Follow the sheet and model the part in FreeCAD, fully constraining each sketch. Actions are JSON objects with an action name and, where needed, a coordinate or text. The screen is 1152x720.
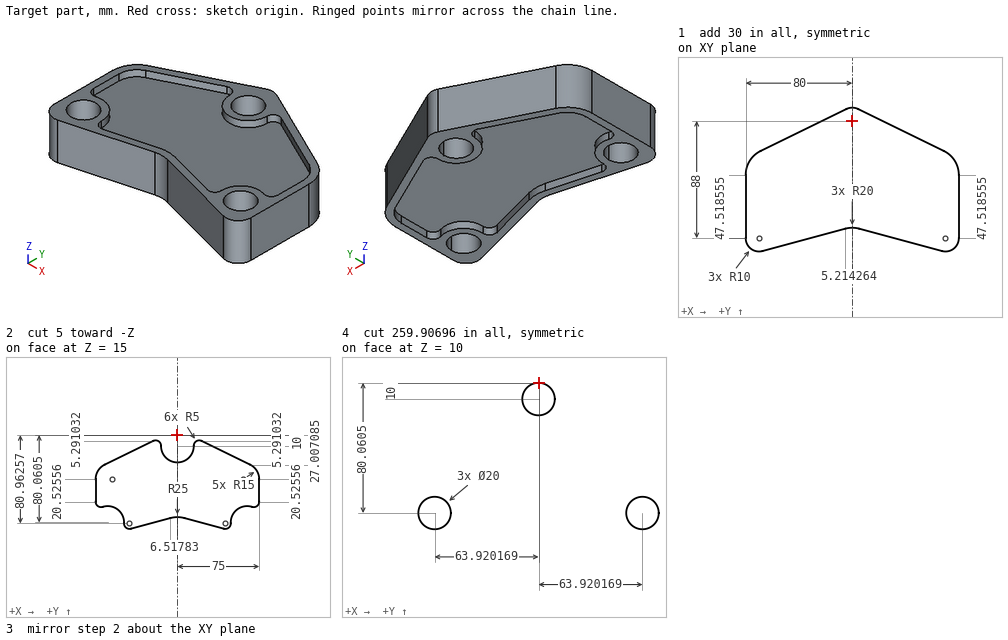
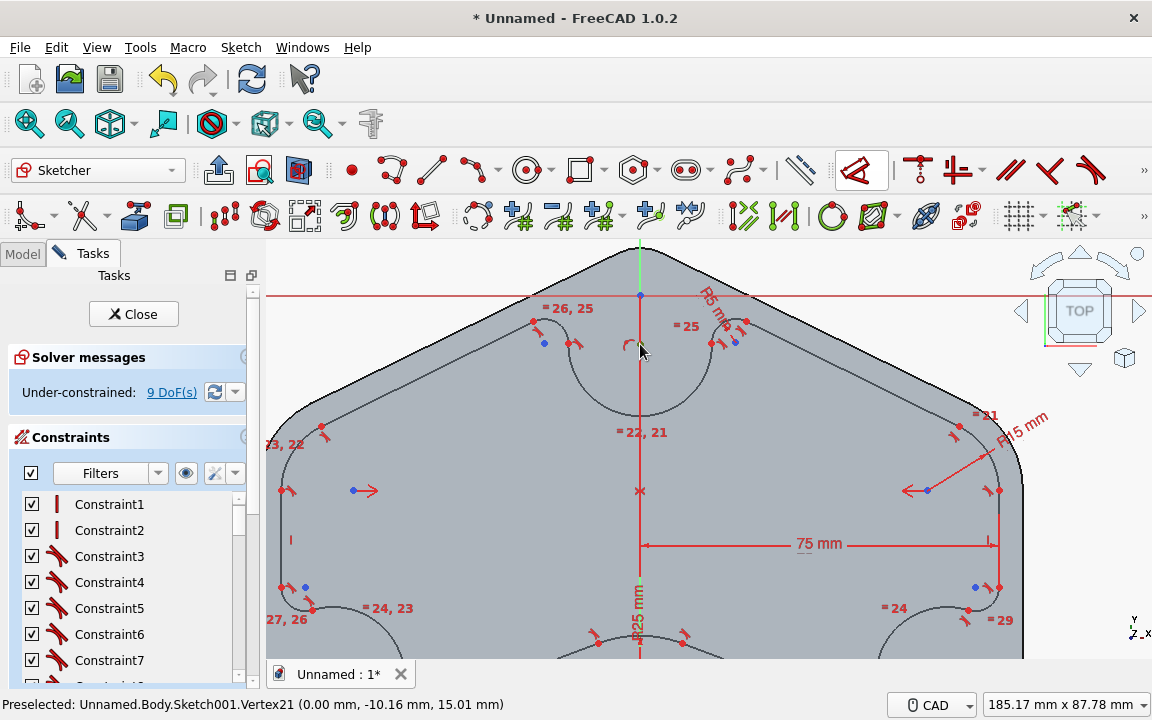
{"action": "left_click", "coordinate": [882, 170]}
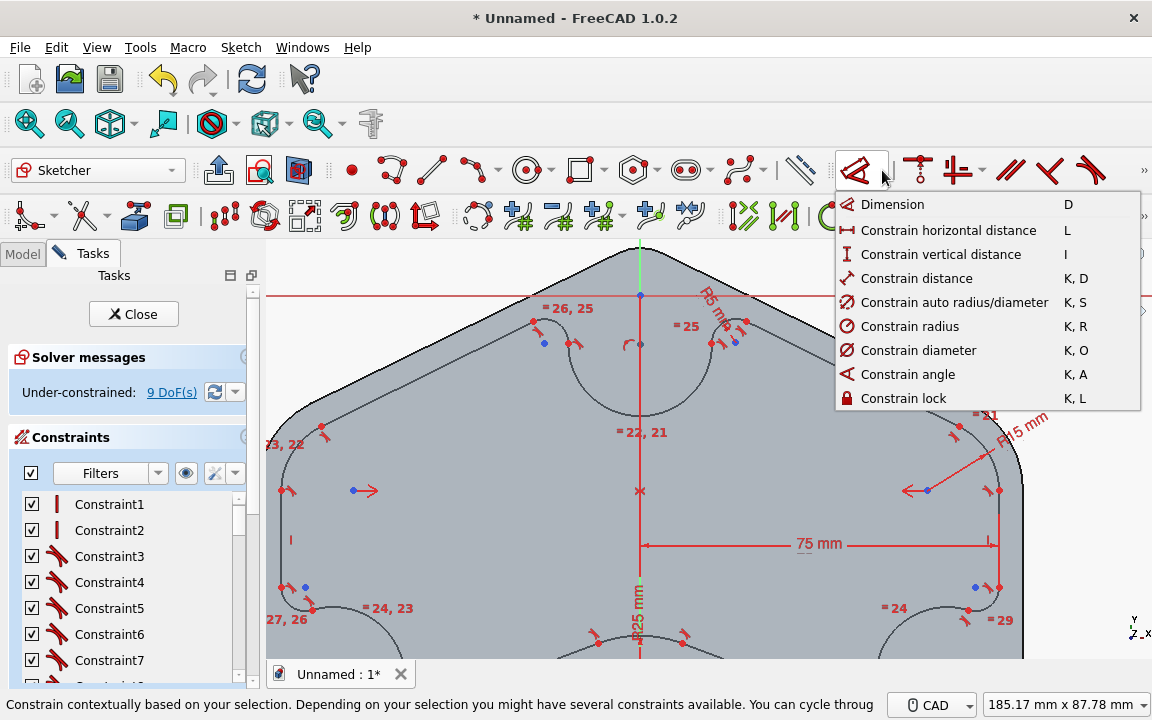
{"action": "left_click", "coordinate": [988, 254]}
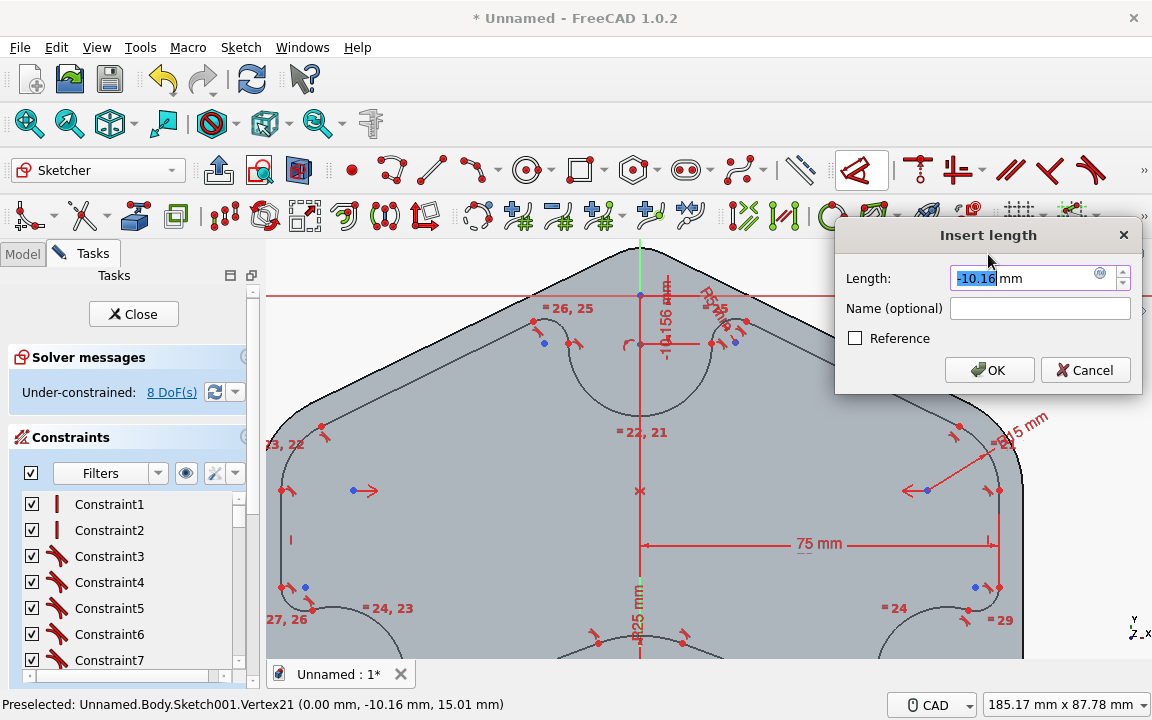
{"action": "type", "text": "-10"}
{"action": "key", "text": "Return"}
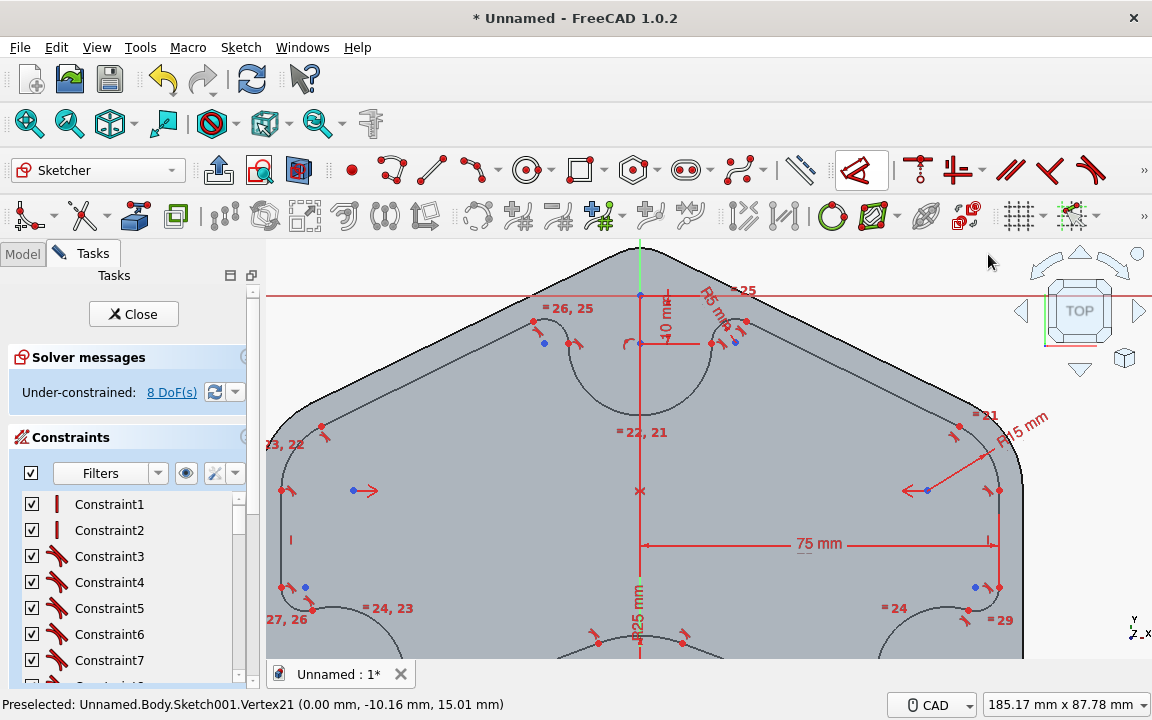
{"action": "scroll", "coordinate": [641, 343], "scroll_direction": "down", "scroll_amount": 2}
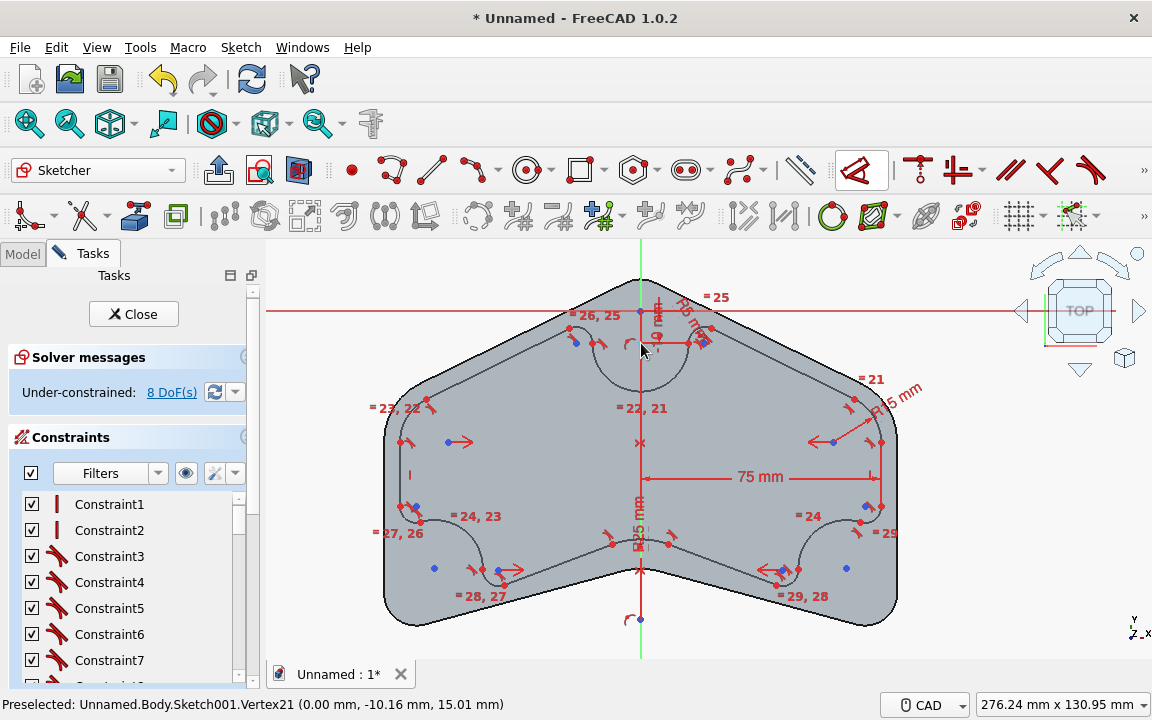
{"action": "left_click", "coordinate": [881, 487]}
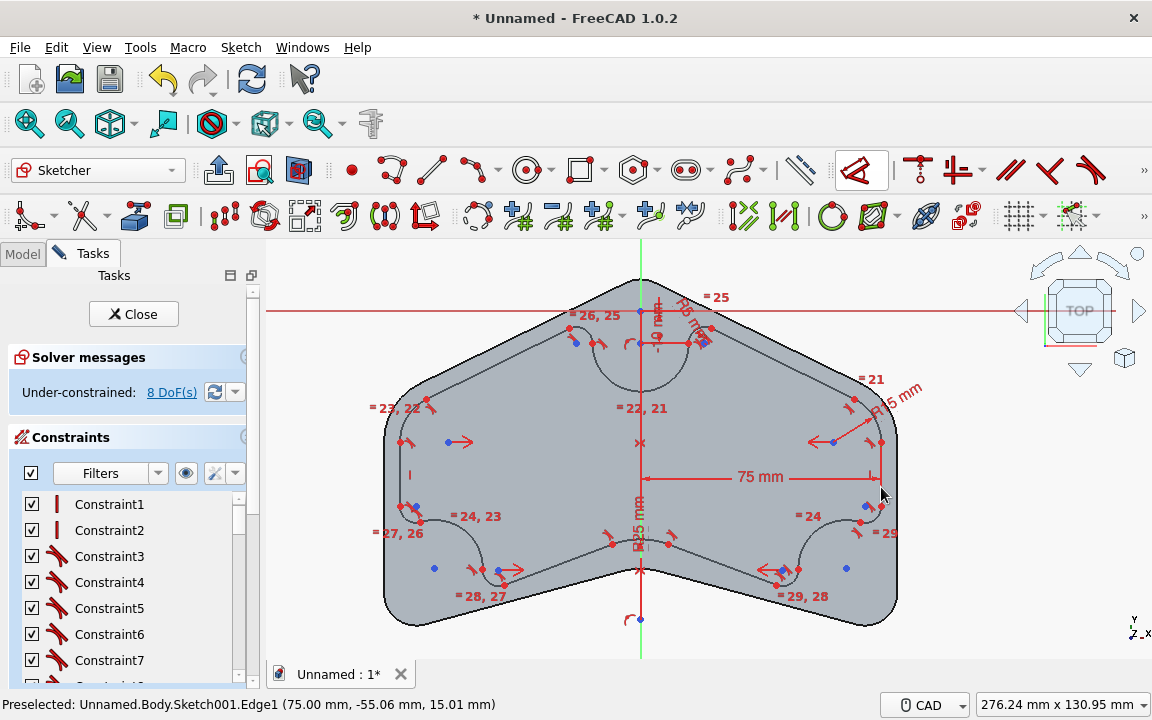
{"action": "key", "text": "i"}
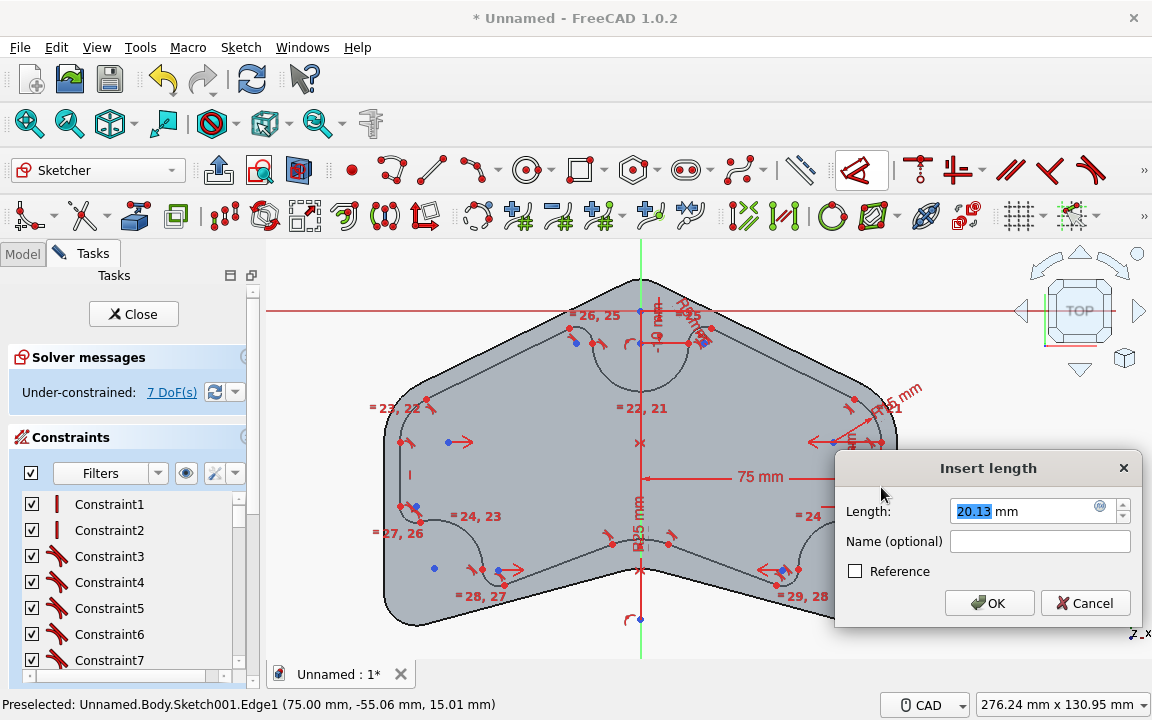
{"action": "type", "text": "20.52556"}
{"action": "key", "text": "Return"}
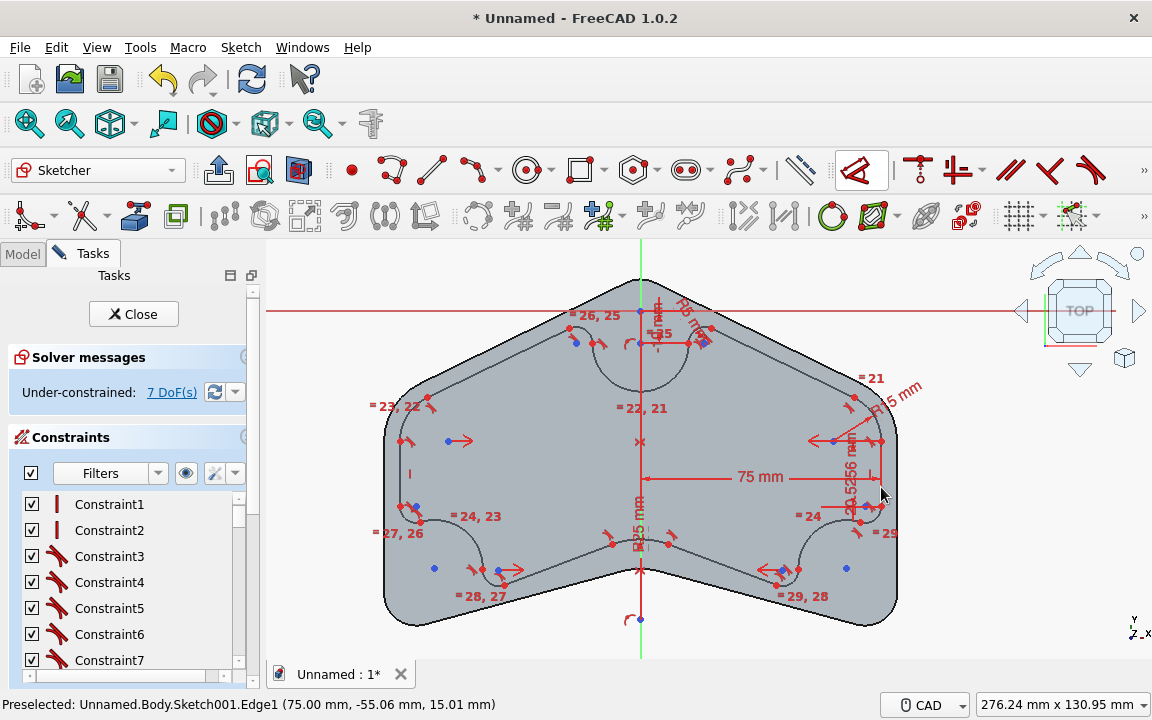
{"action": "left_click", "coordinate": [400, 461]}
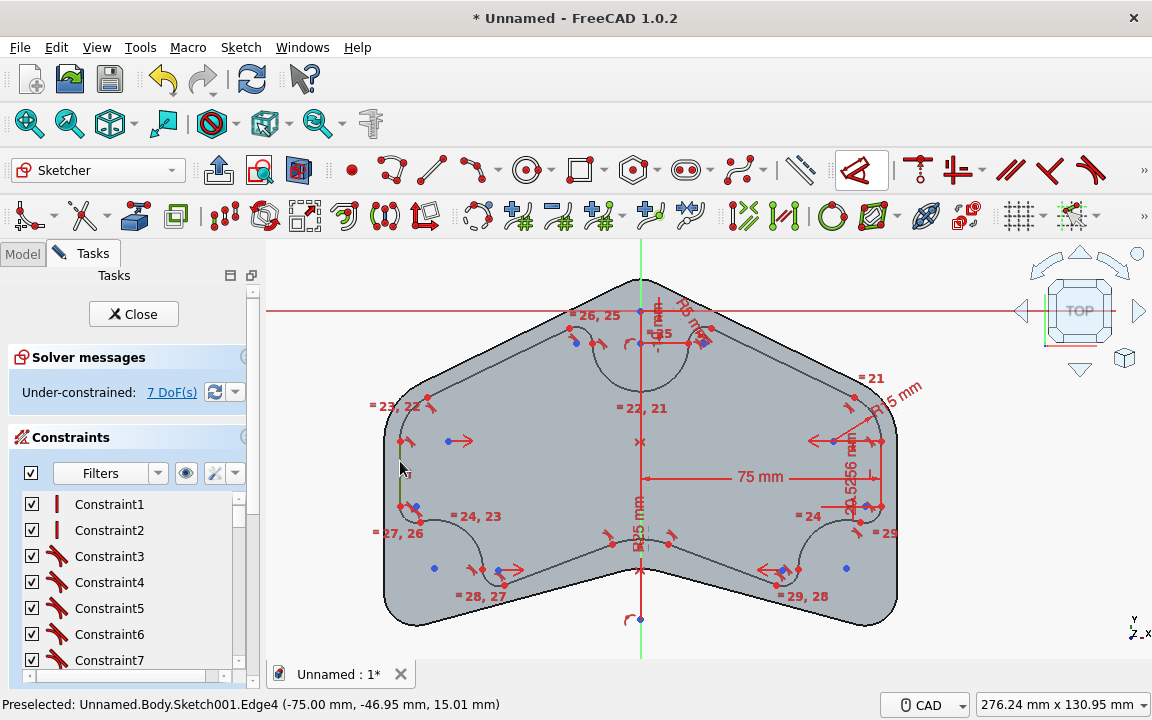
{"action": "left_click", "coordinate": [882, 170]}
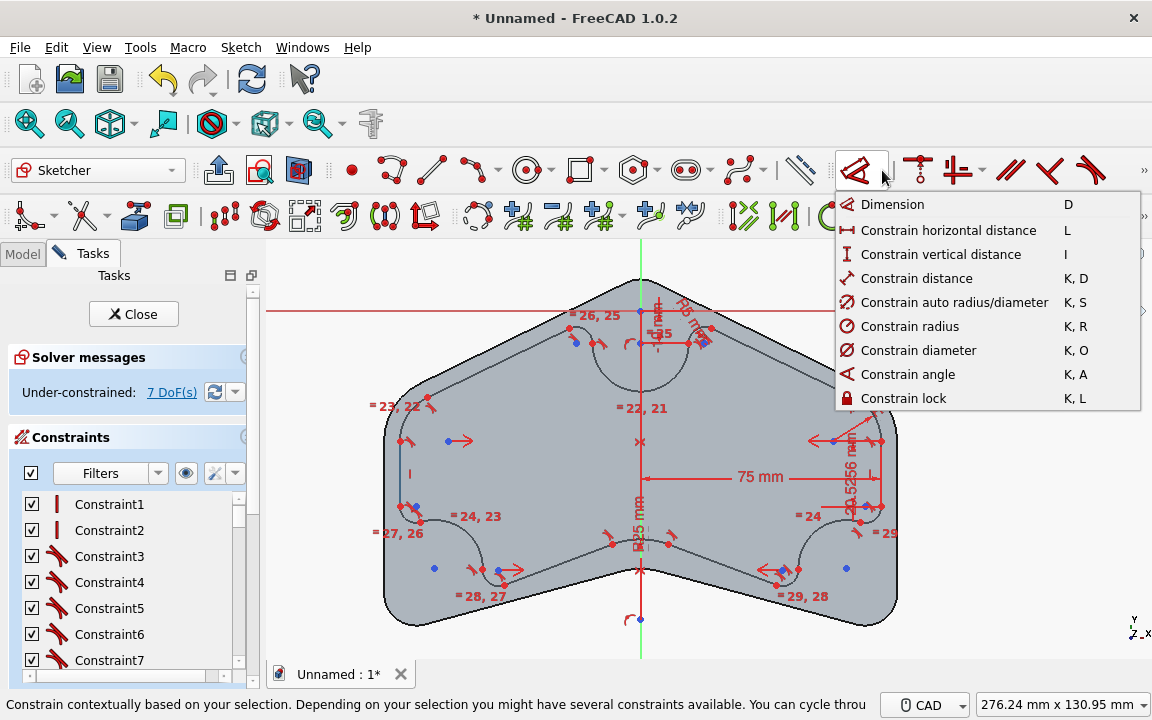
{"action": "left_click", "coordinate": [988, 254]}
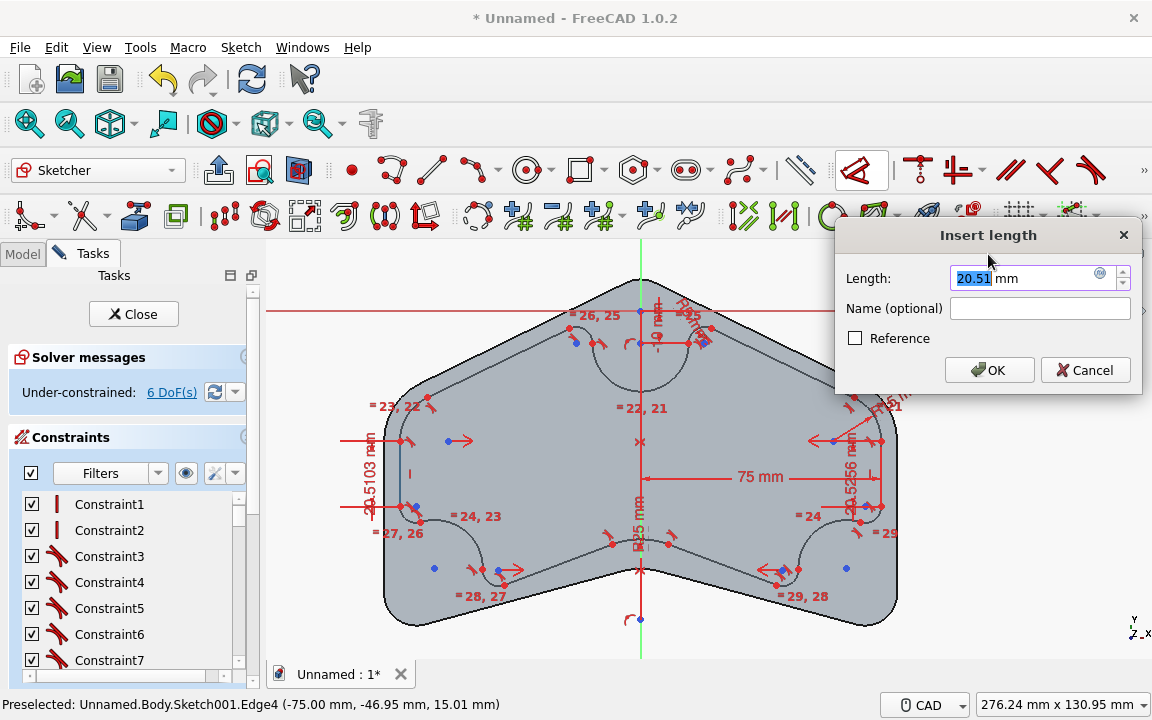
{"action": "type", "text": "20.52556"}
{"action": "key", "text": "Return"}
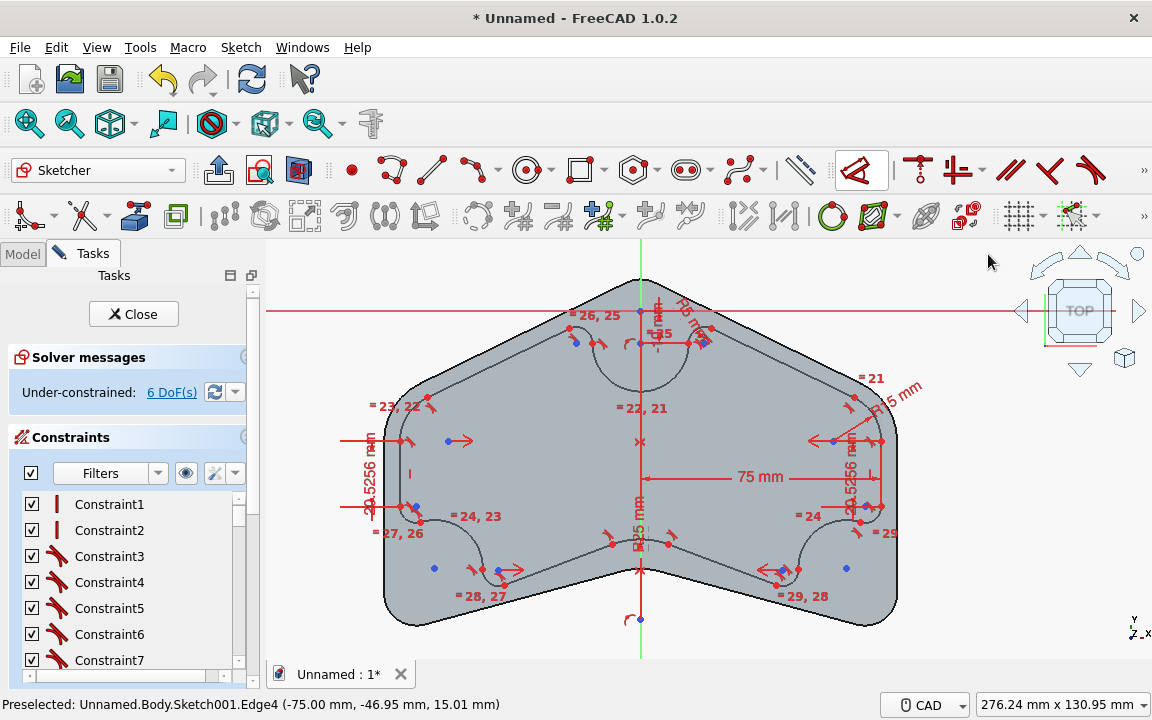
{"action": "scroll", "coordinate": [612, 544], "scroll_direction": "up", "scroll_amount": 4}